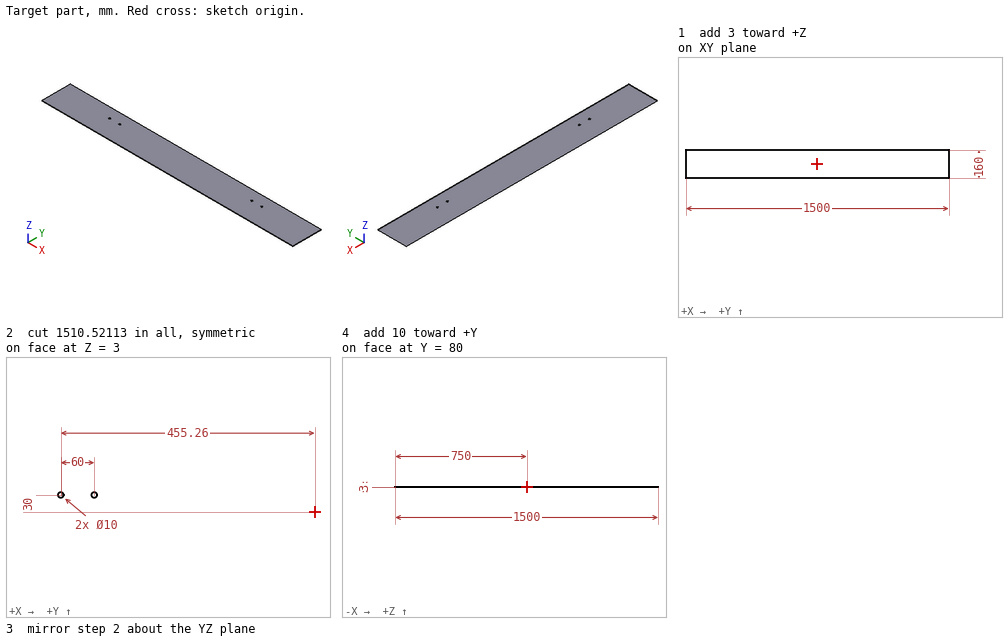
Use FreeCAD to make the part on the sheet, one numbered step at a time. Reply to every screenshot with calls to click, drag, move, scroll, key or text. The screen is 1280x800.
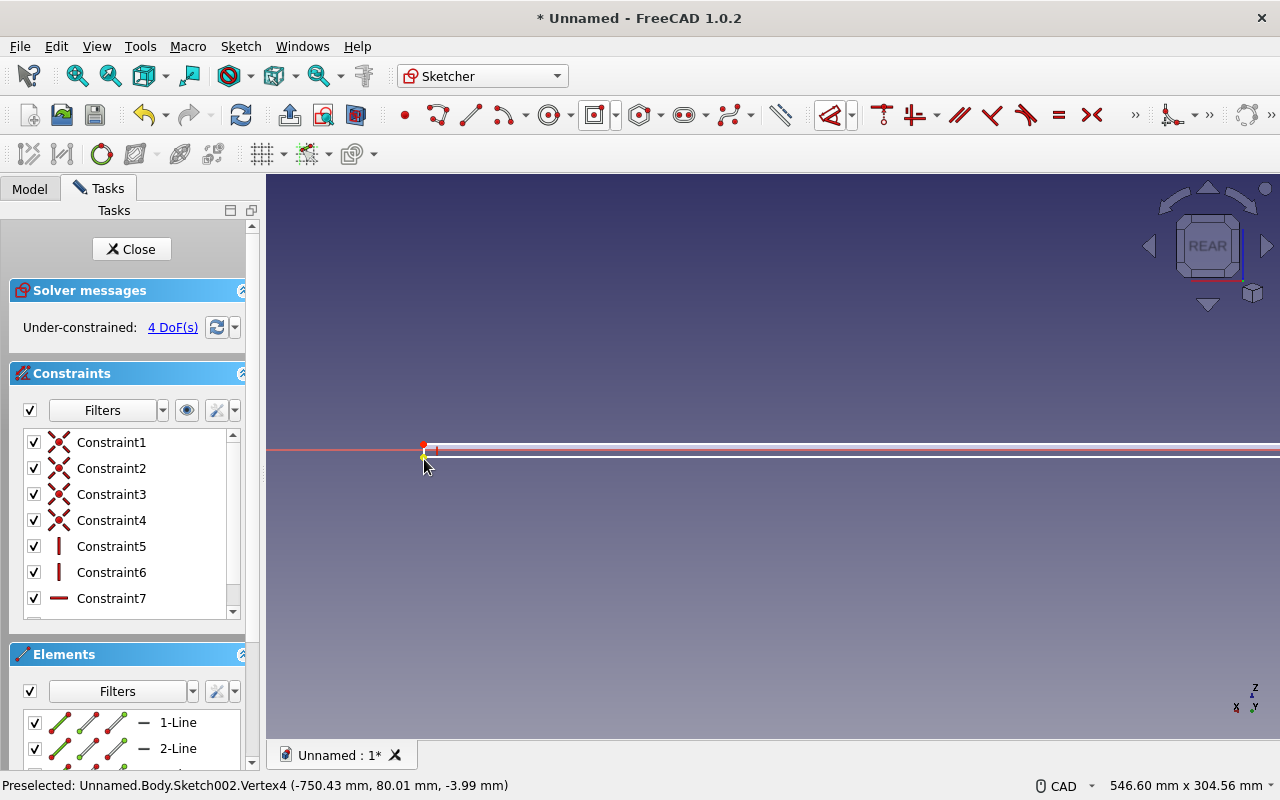
click(424, 457)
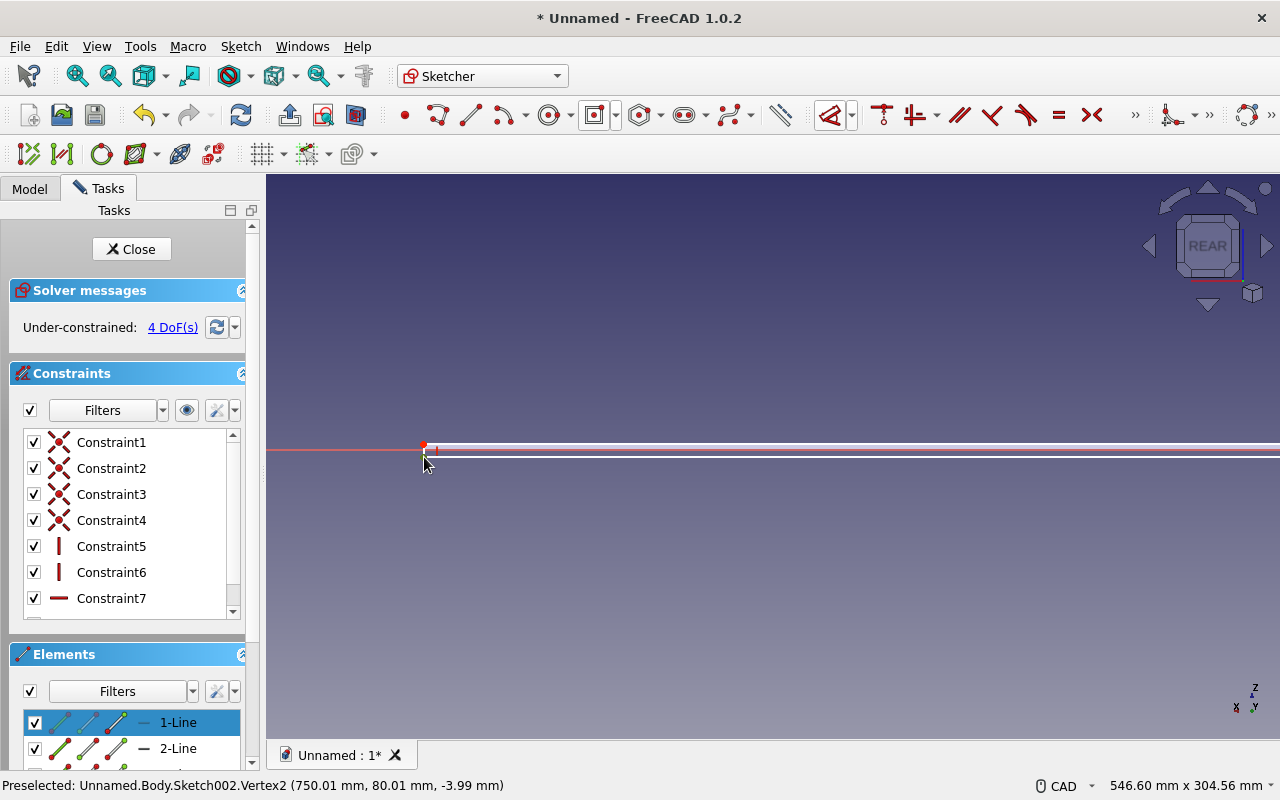
click(353, 450)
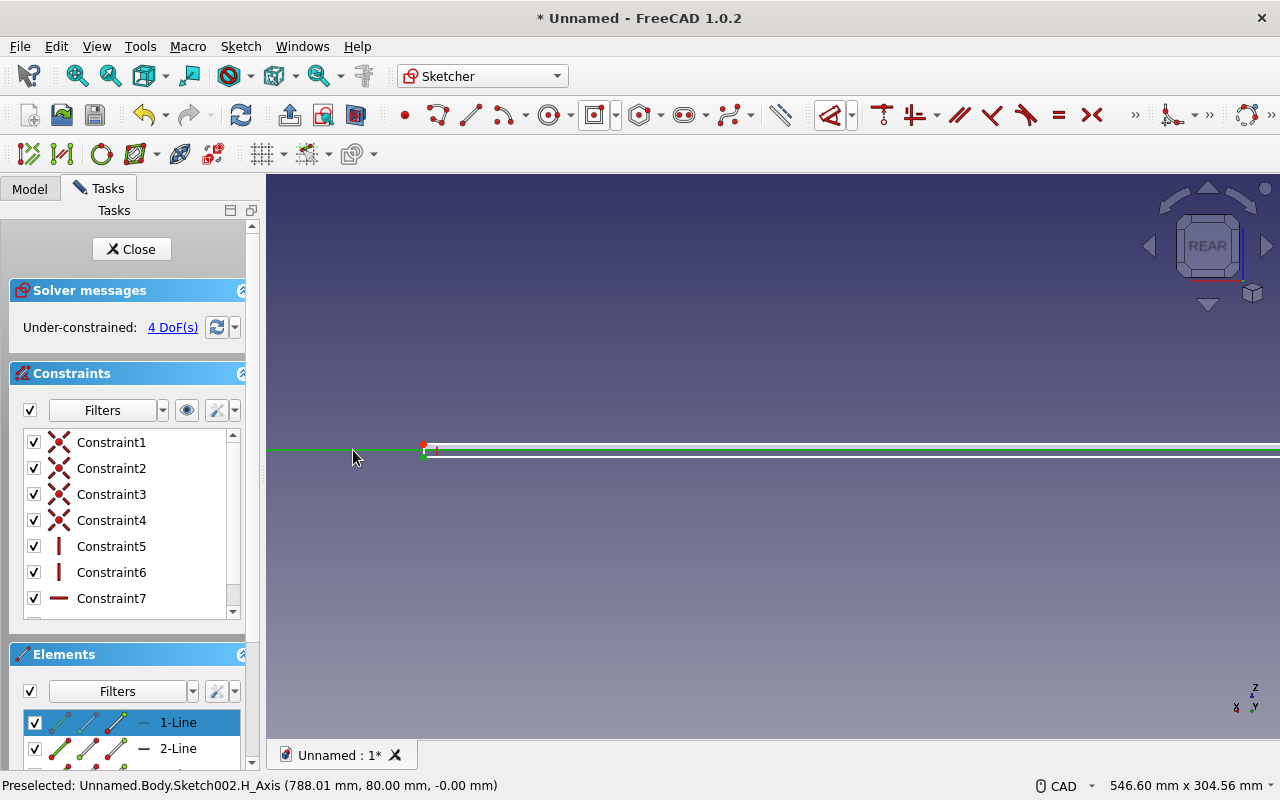
click(882, 116)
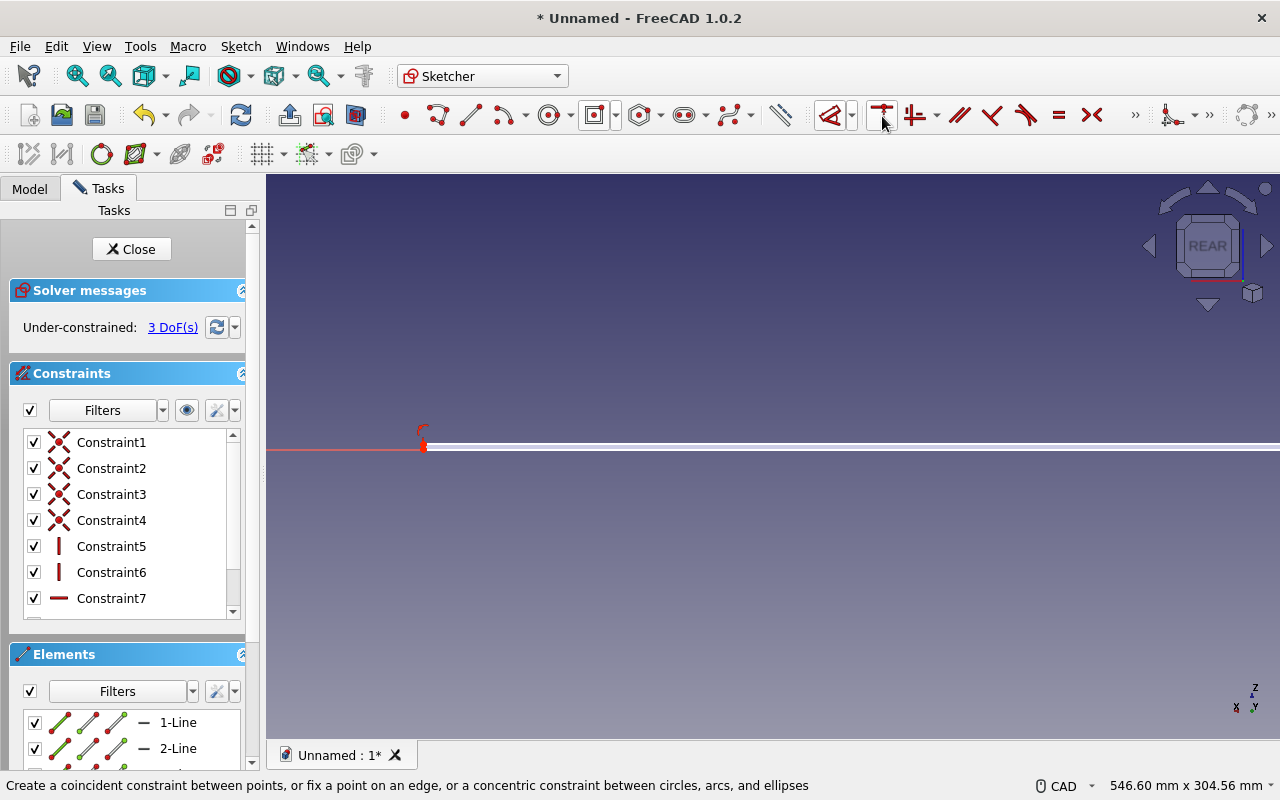
scroll(424, 447, up, 10)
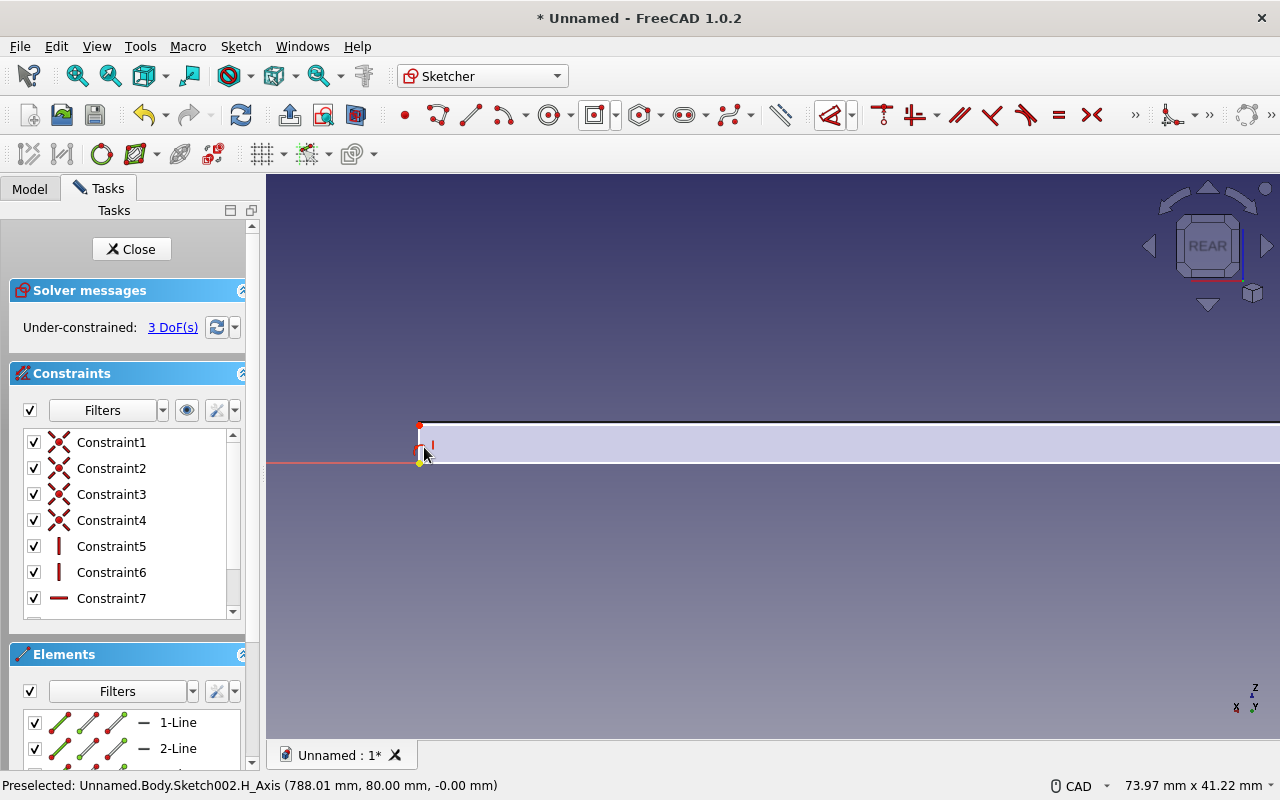
click(419, 440)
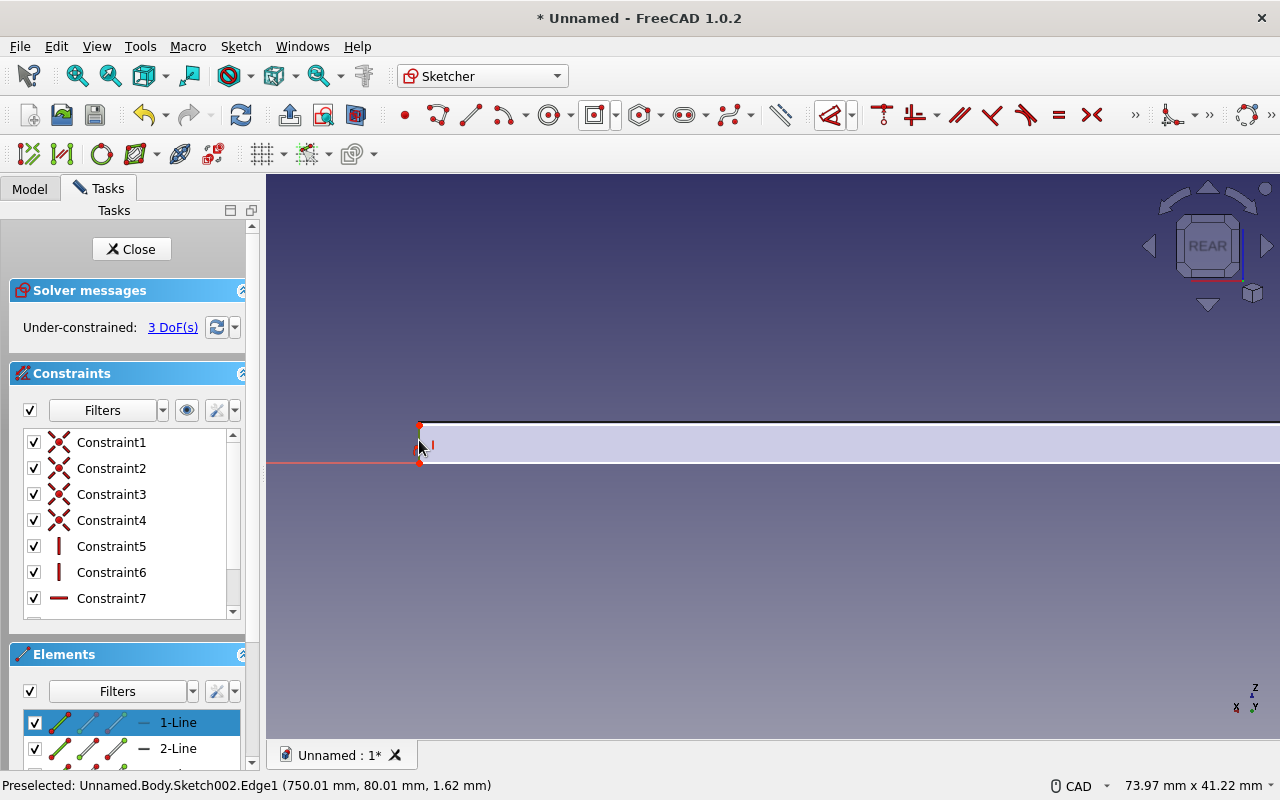
key(i)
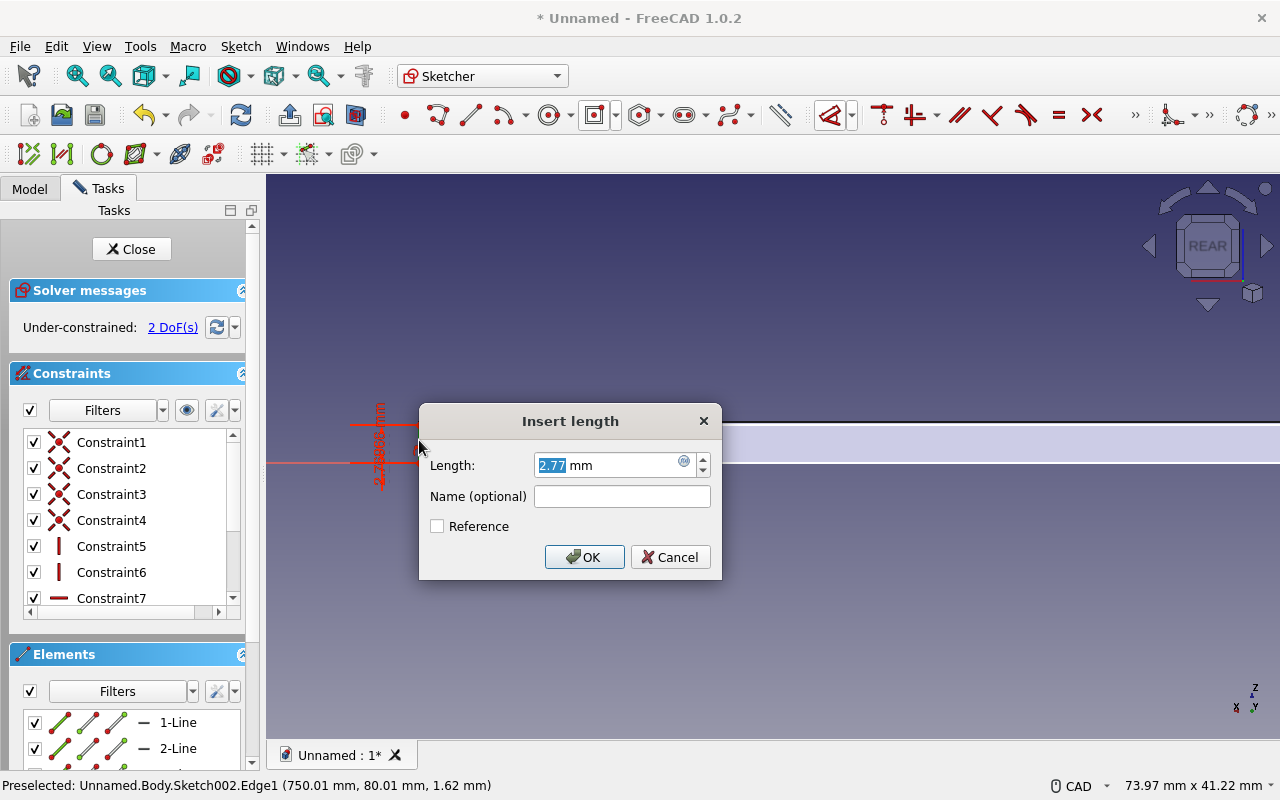
text(3)
key(Return)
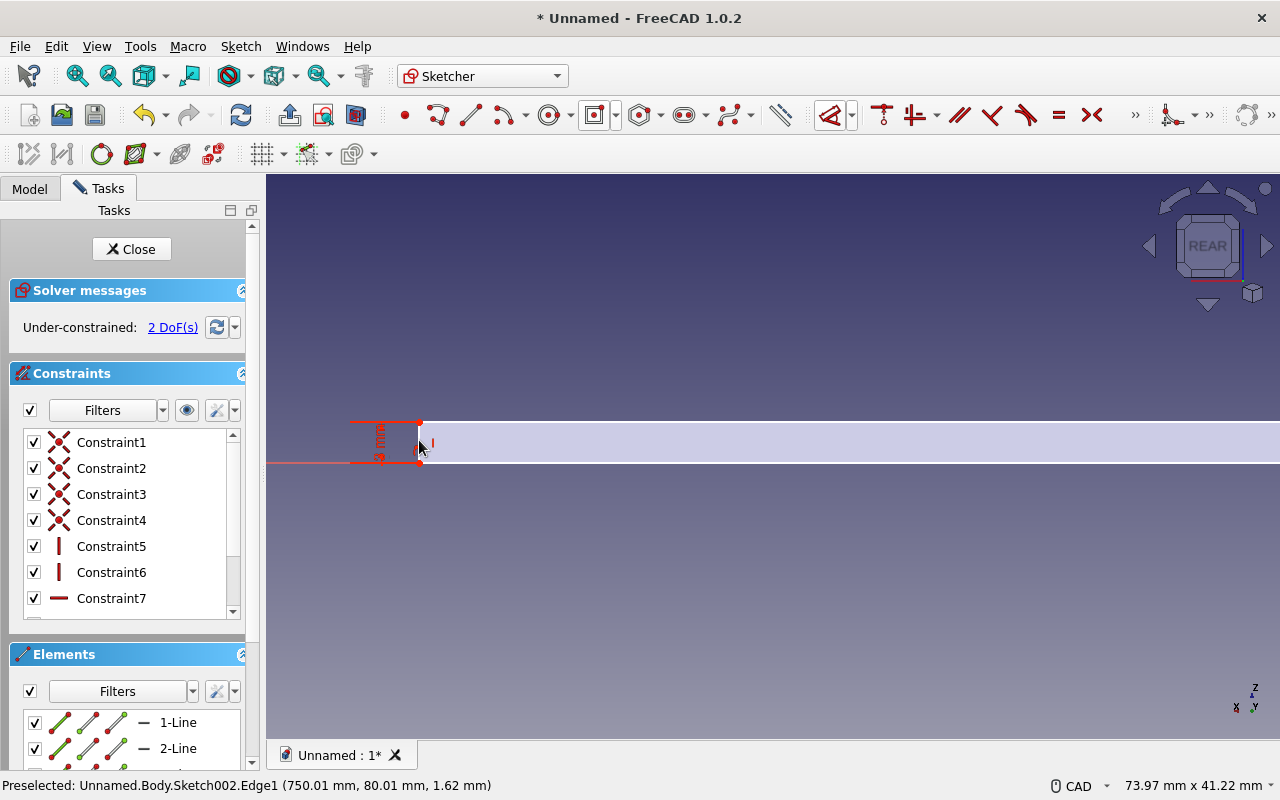
scroll(359, 457, down, 17)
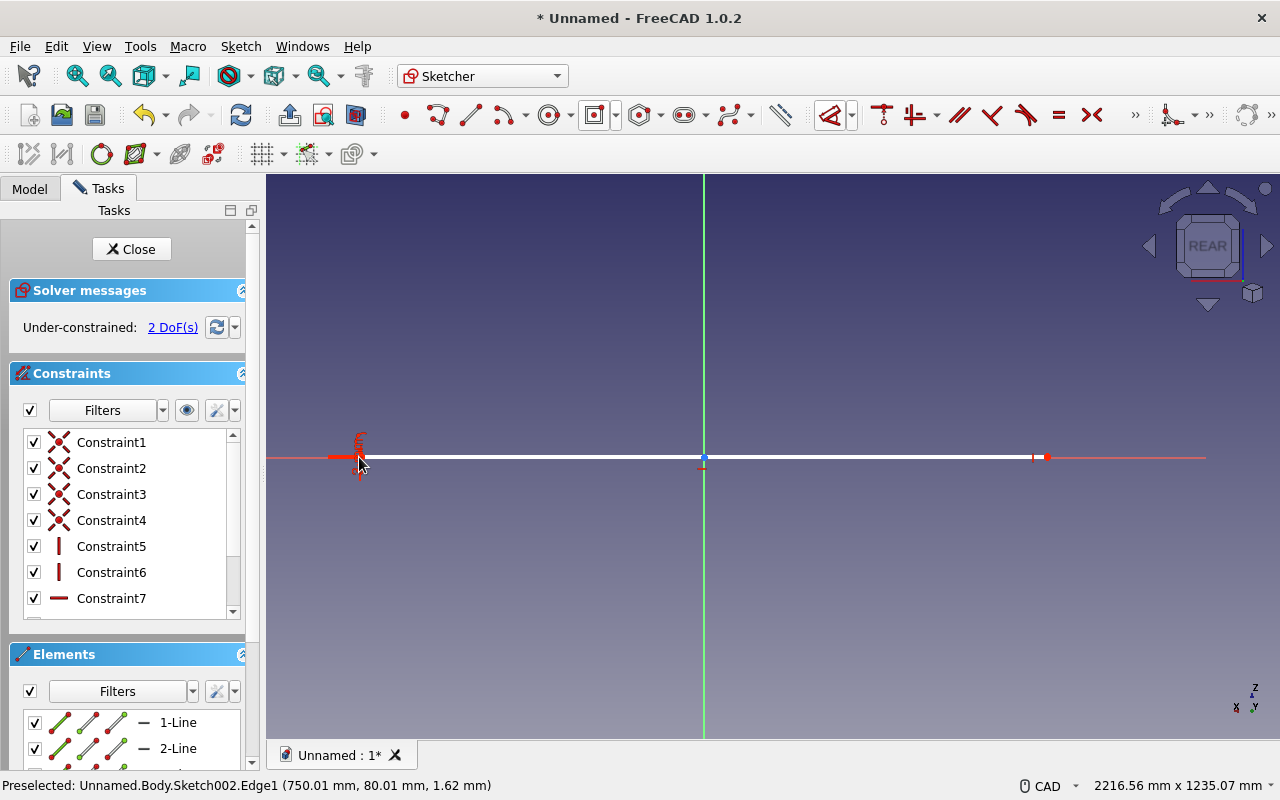
scroll(567, 458, up, 12)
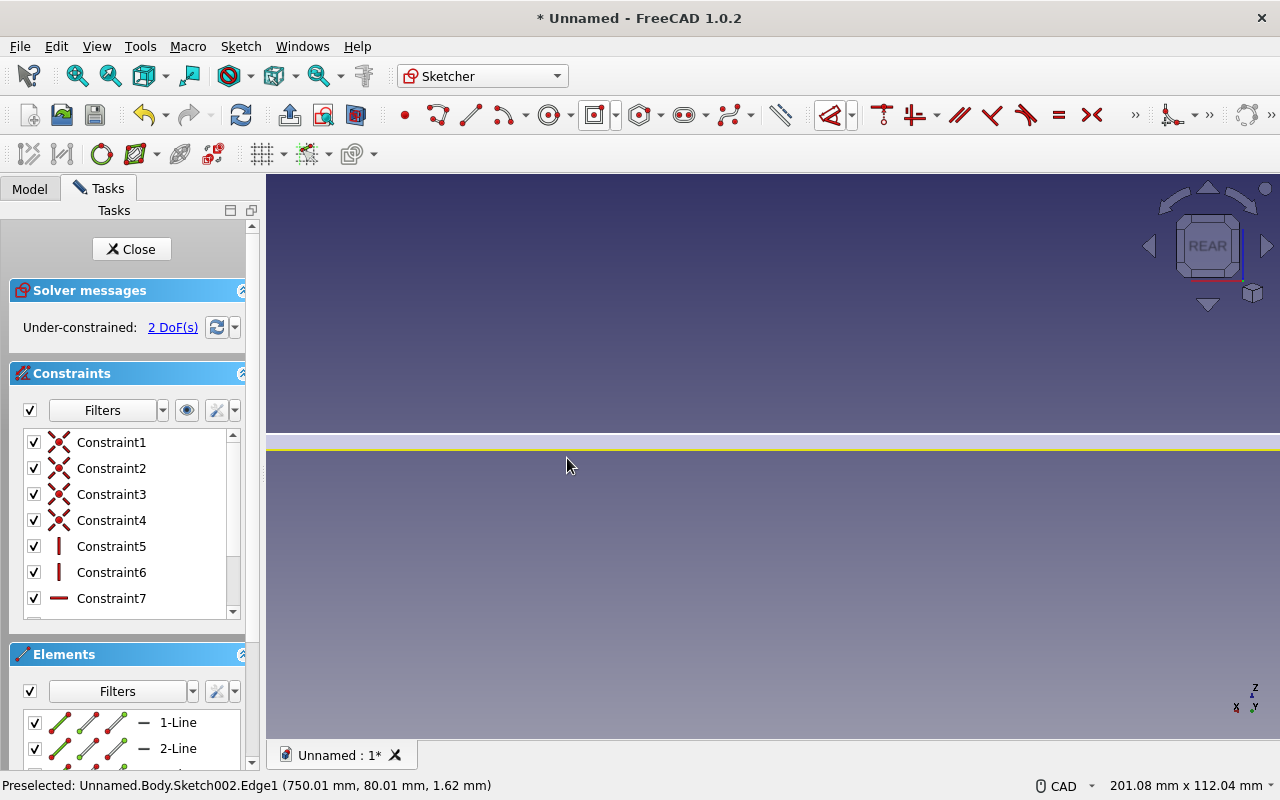
click(564, 450)